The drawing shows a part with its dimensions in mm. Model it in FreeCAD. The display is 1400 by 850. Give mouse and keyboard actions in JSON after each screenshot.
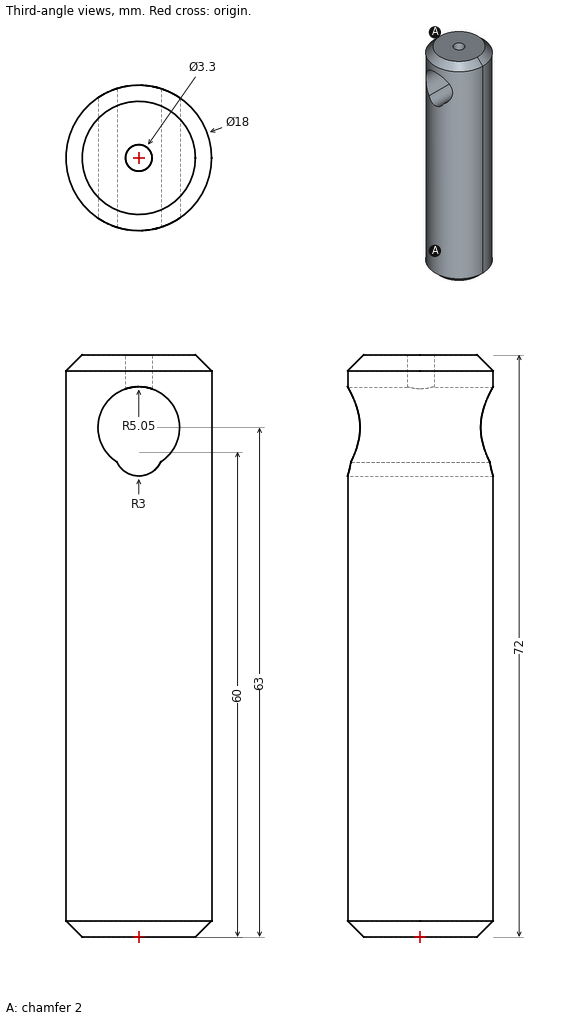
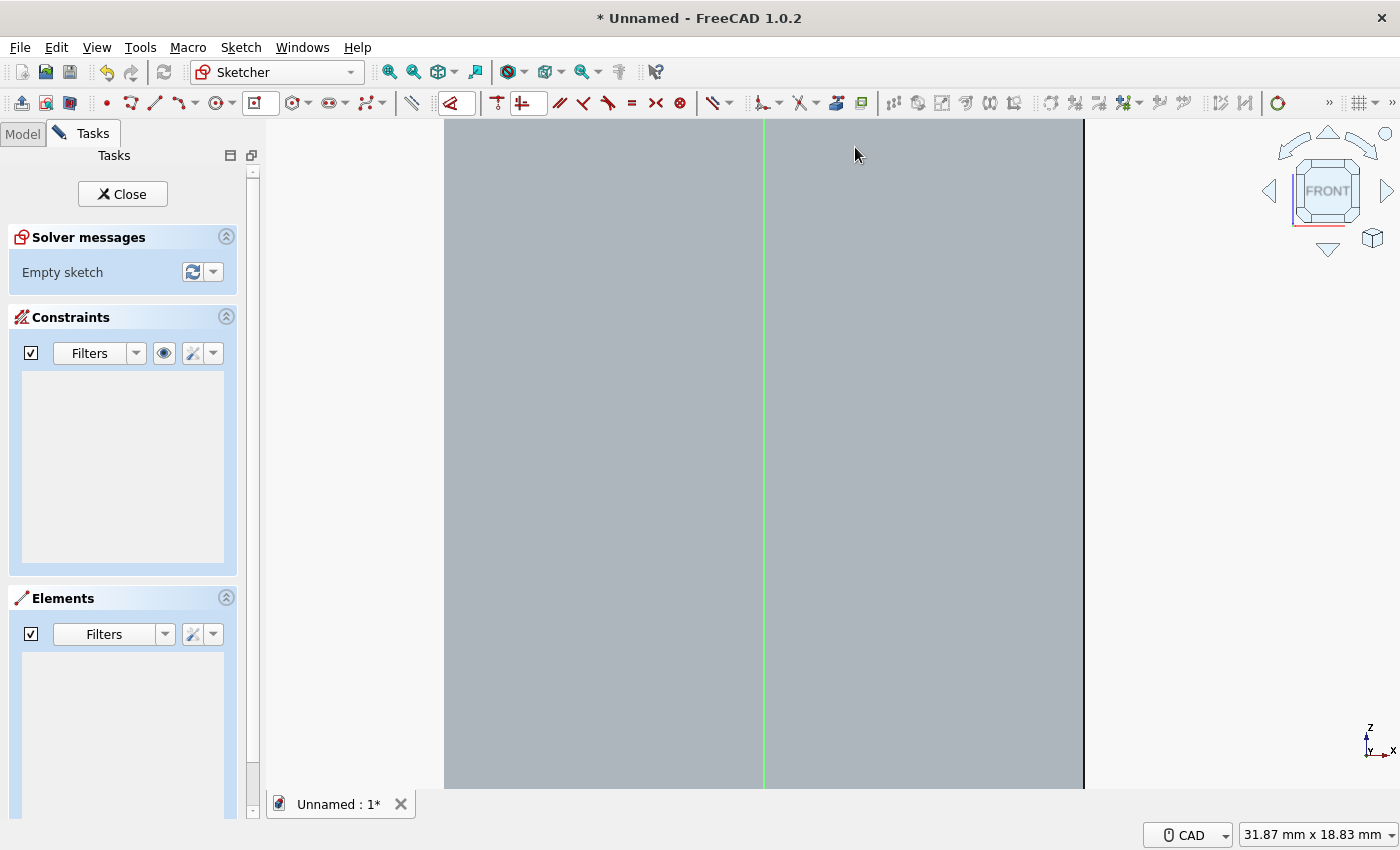
{"action": "left_click", "coordinate": [180, 104]}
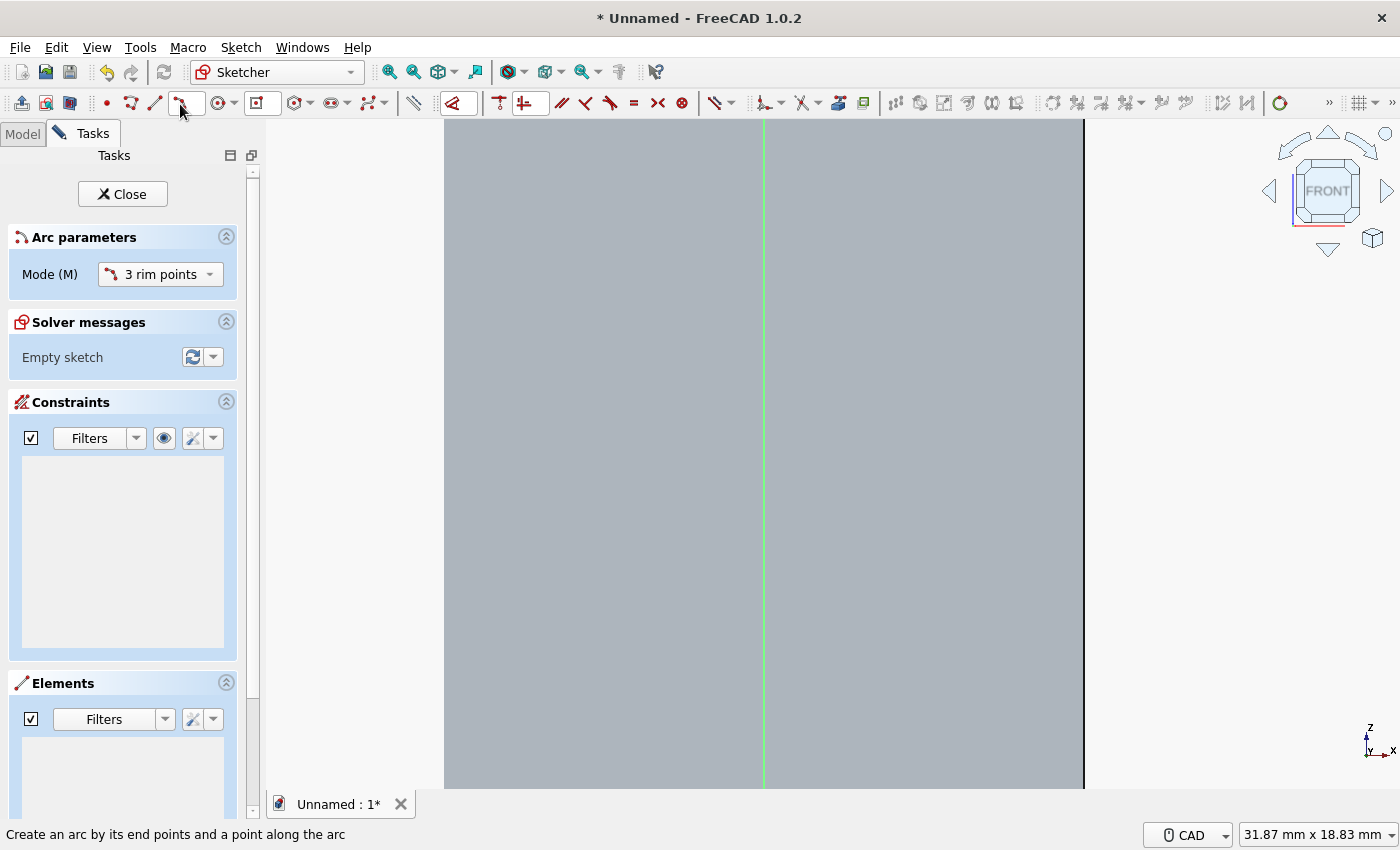
{"action": "left_click", "coordinate": [861, 582]}
{"action": "left_click", "coordinate": [667, 582]}
{"action": "left_click", "coordinate": [853, 275]}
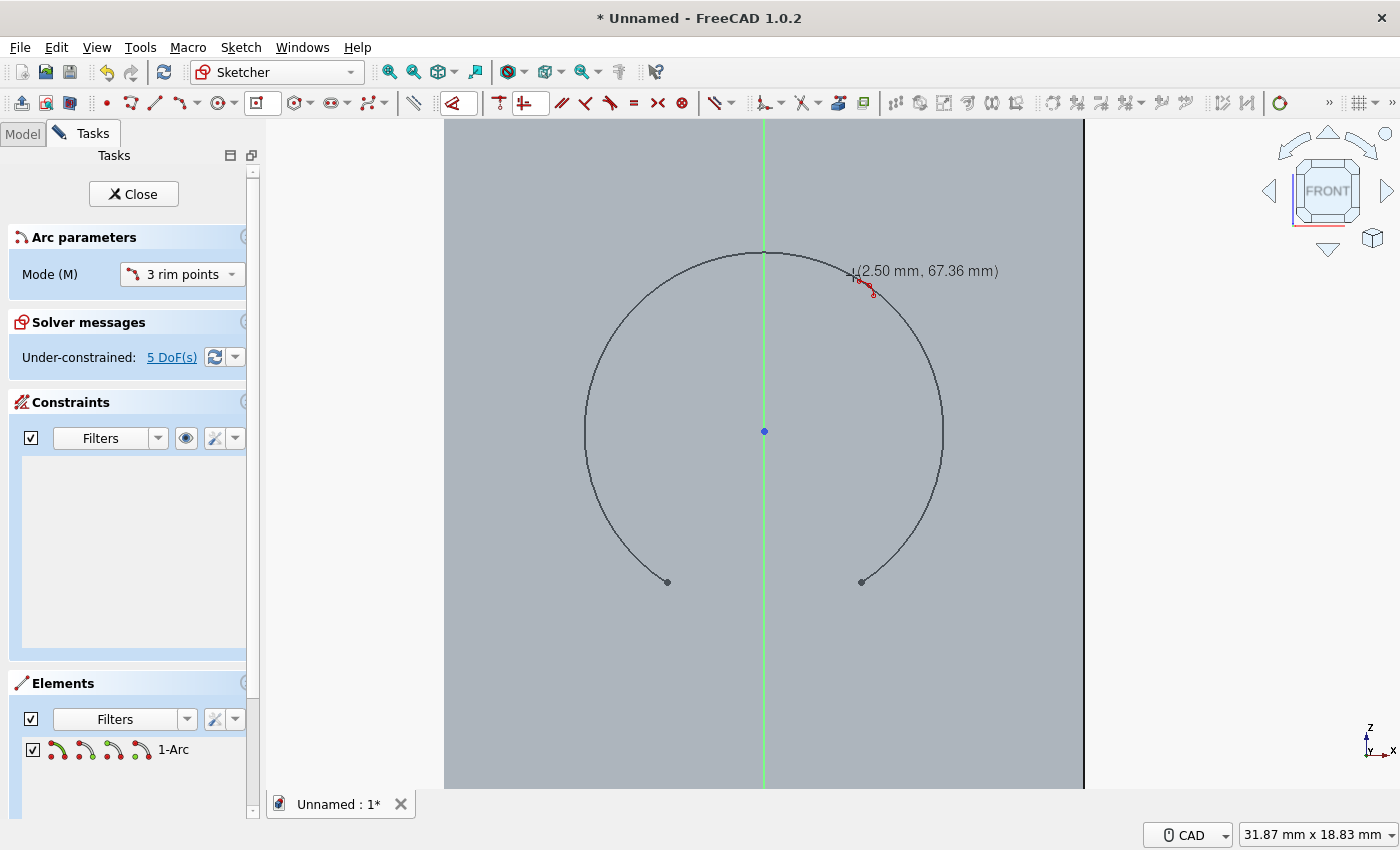
{"action": "left_click", "coordinate": [667, 583]}
{"action": "left_click", "coordinate": [861, 583]}
{"action": "left_click", "coordinate": [740, 642]}
{"action": "key", "text": "Escape"}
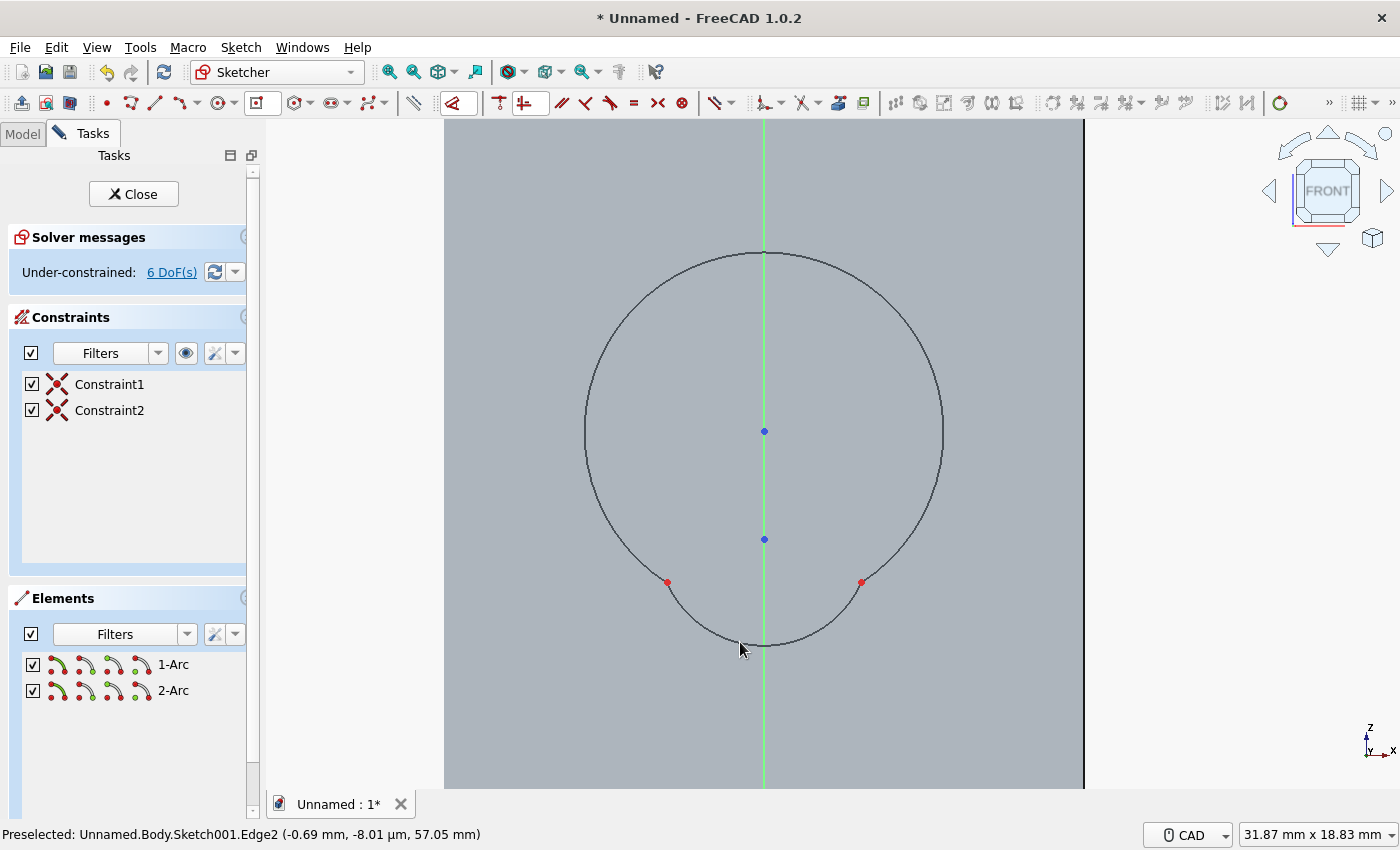
{"action": "left_click", "coordinate": [764, 432]}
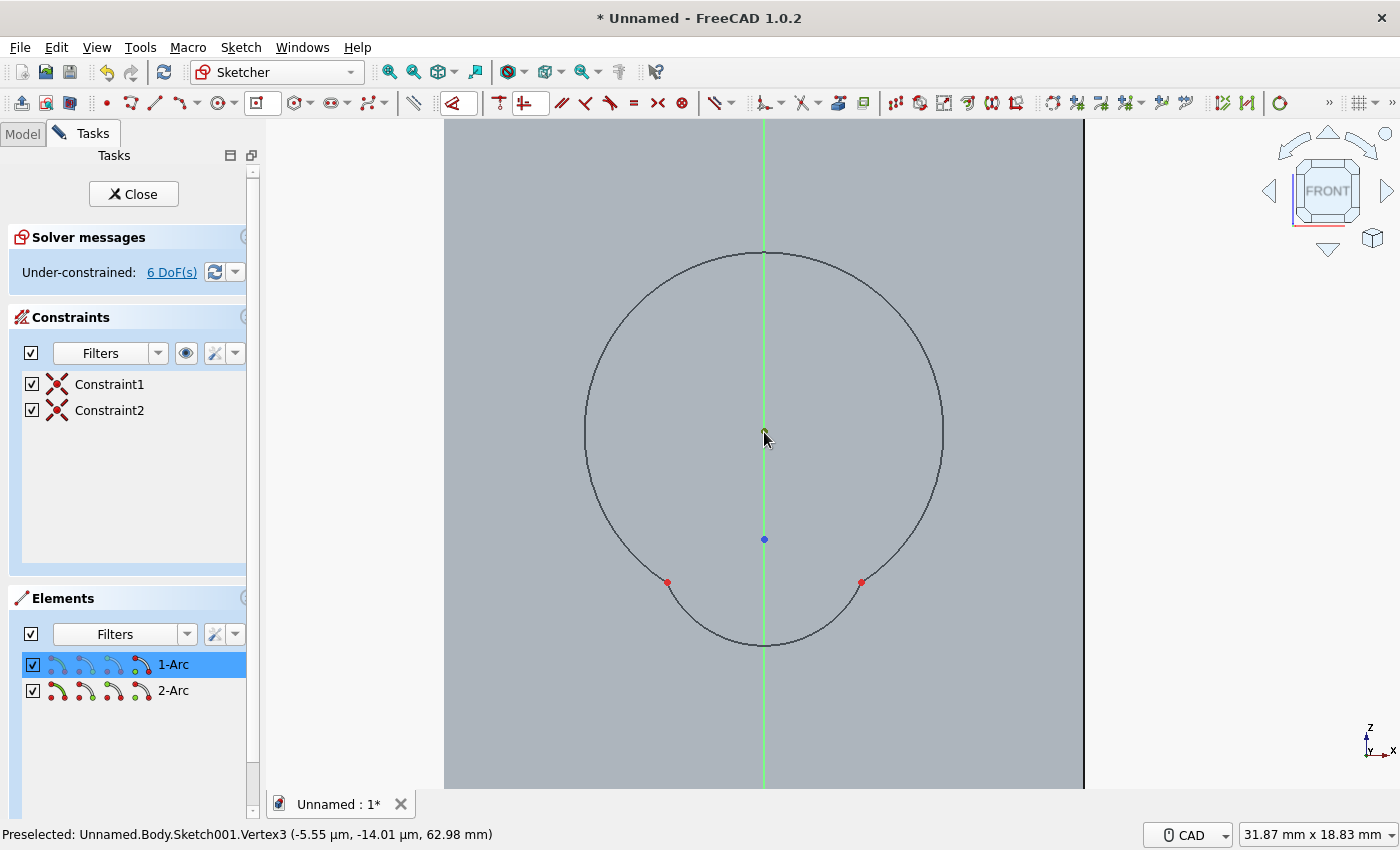
{"action": "left_click", "coordinate": [764, 717]}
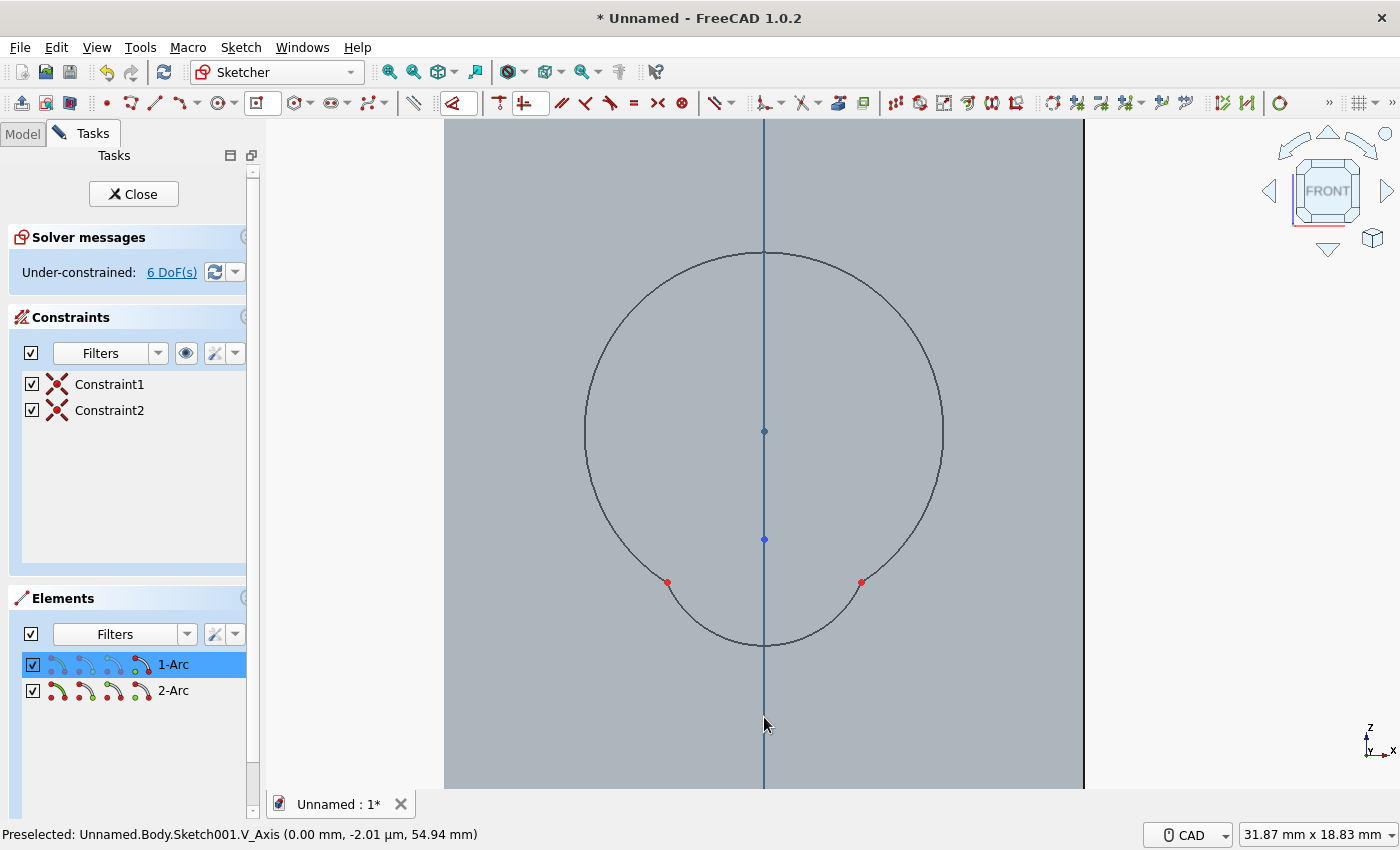
{"action": "left_click", "coordinate": [500, 104]}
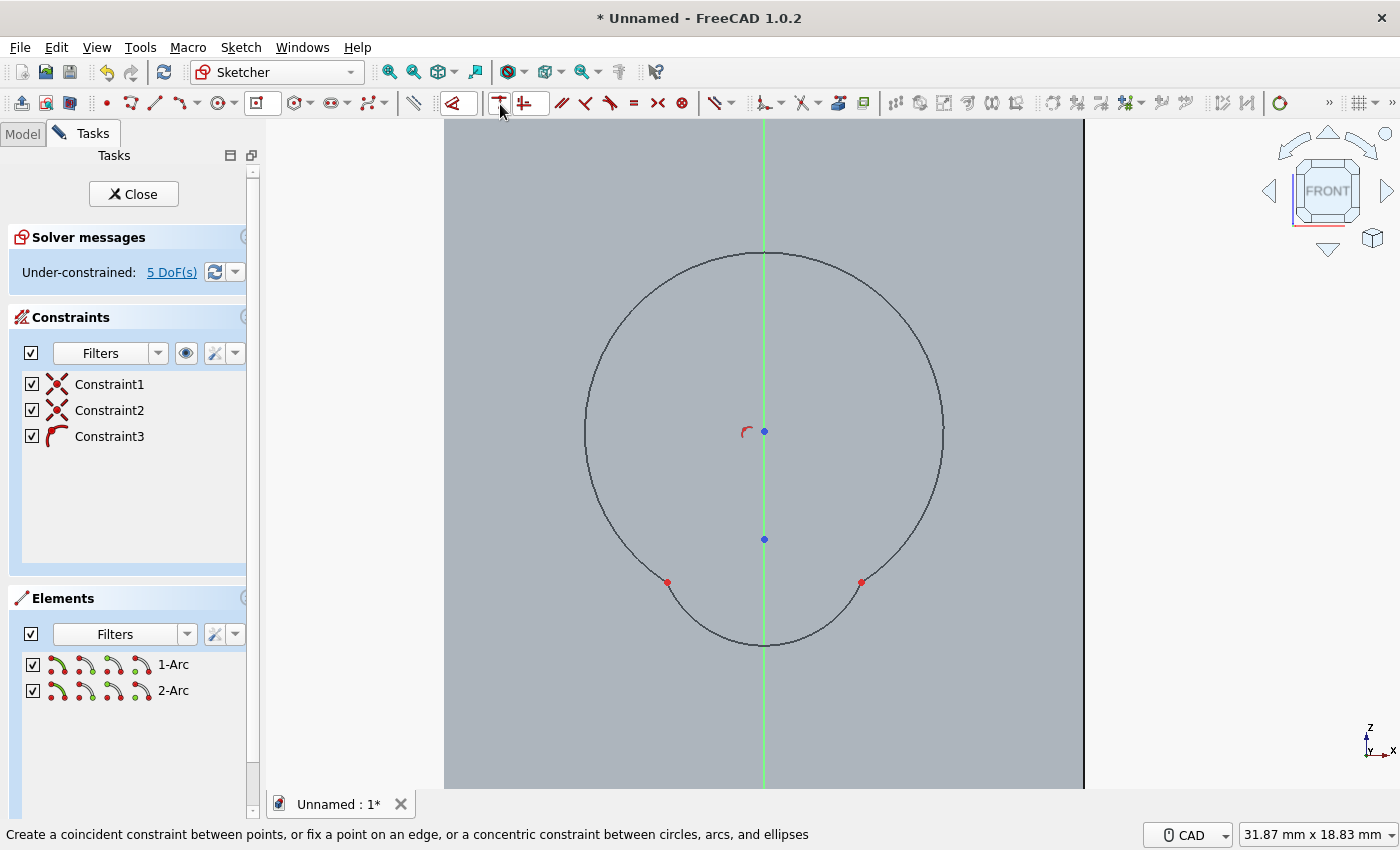
{"action": "left_click", "coordinate": [764, 539]}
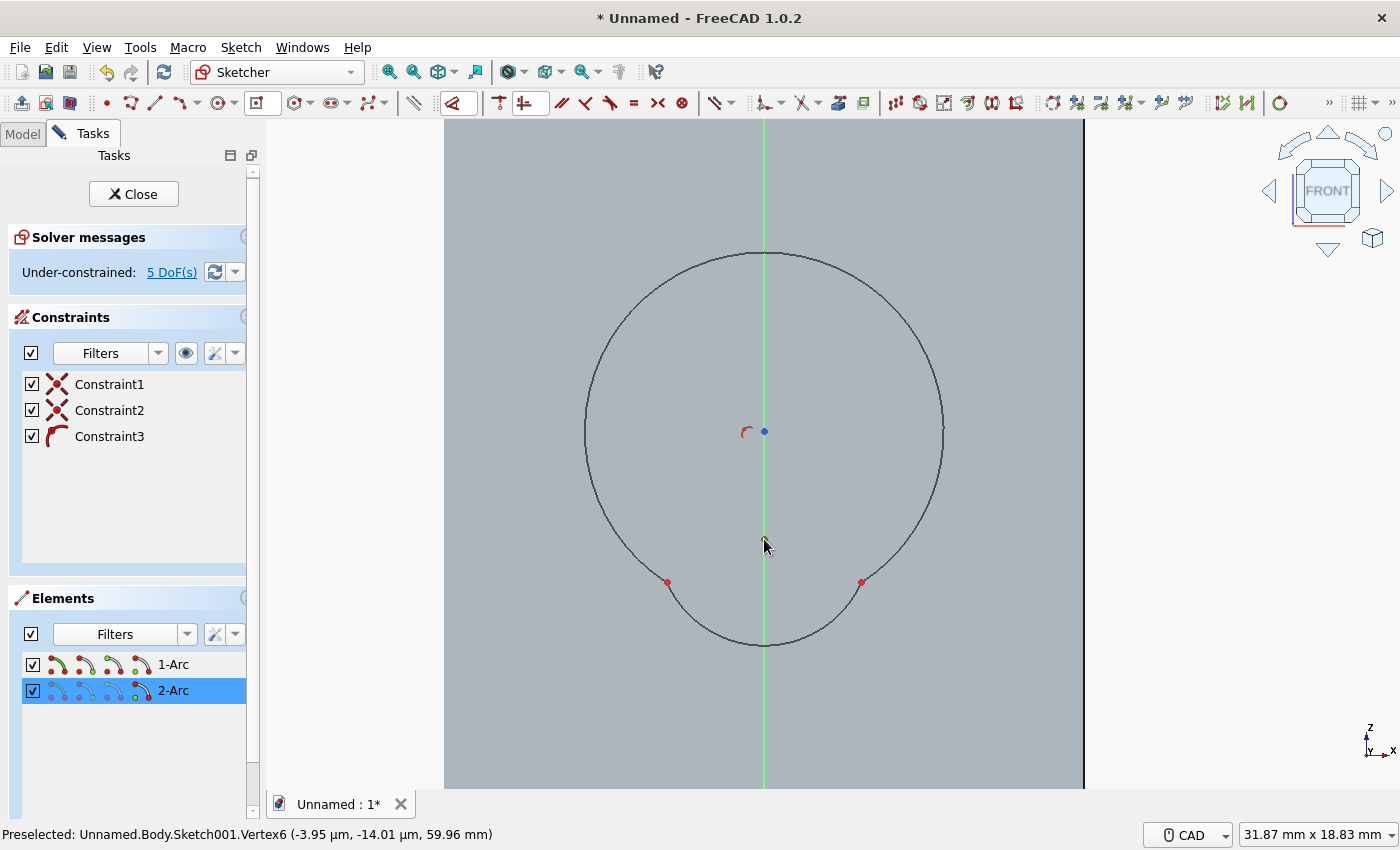
{"action": "left_click", "coordinate": [764, 717]}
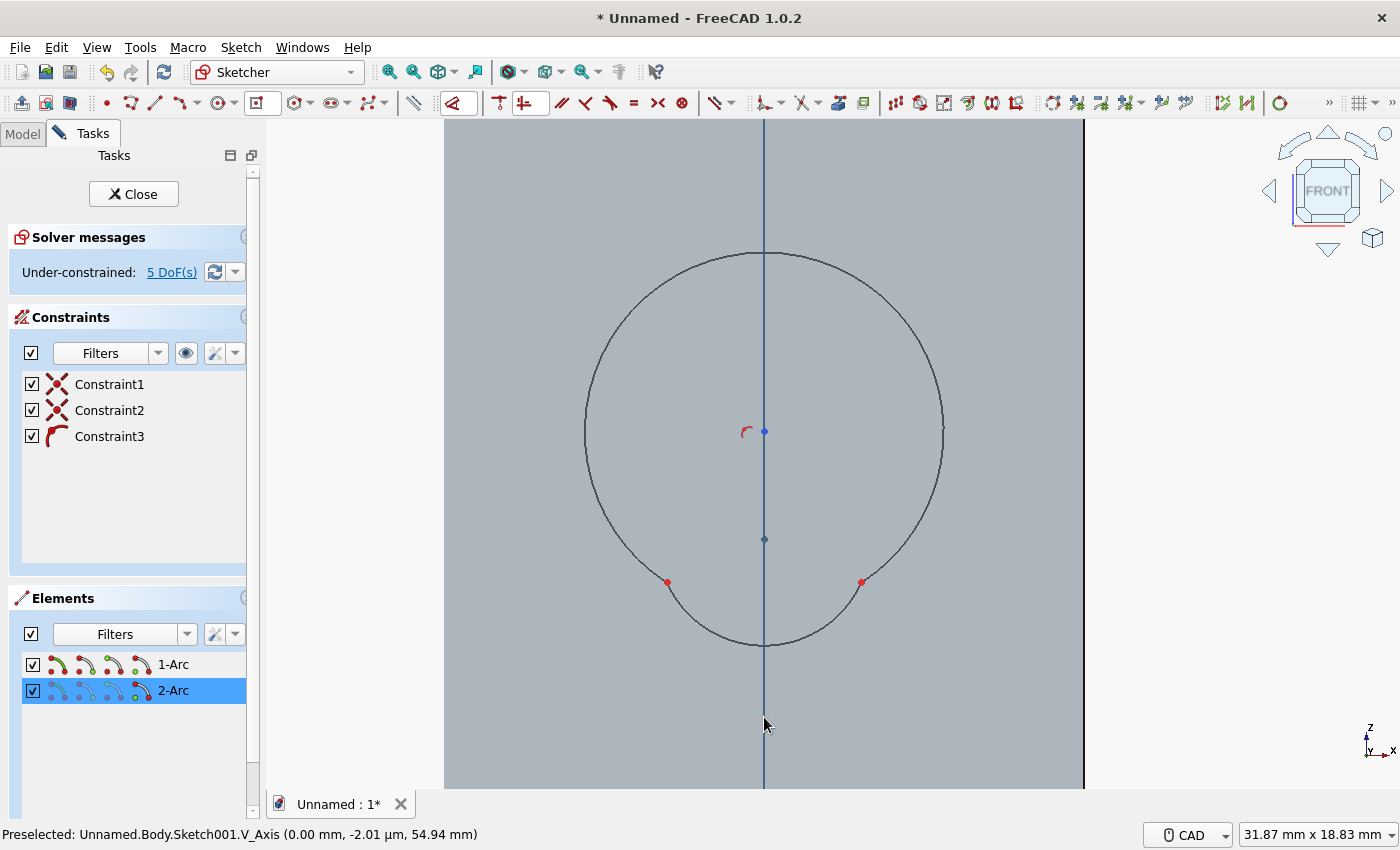
{"action": "key", "text": "c"}